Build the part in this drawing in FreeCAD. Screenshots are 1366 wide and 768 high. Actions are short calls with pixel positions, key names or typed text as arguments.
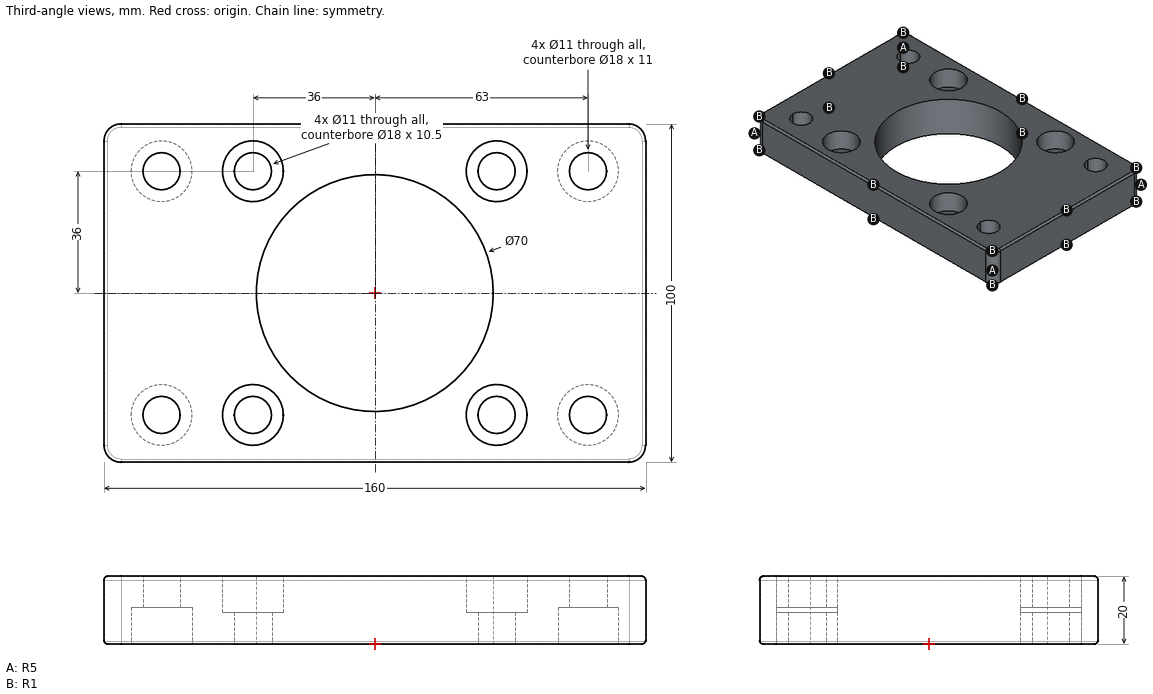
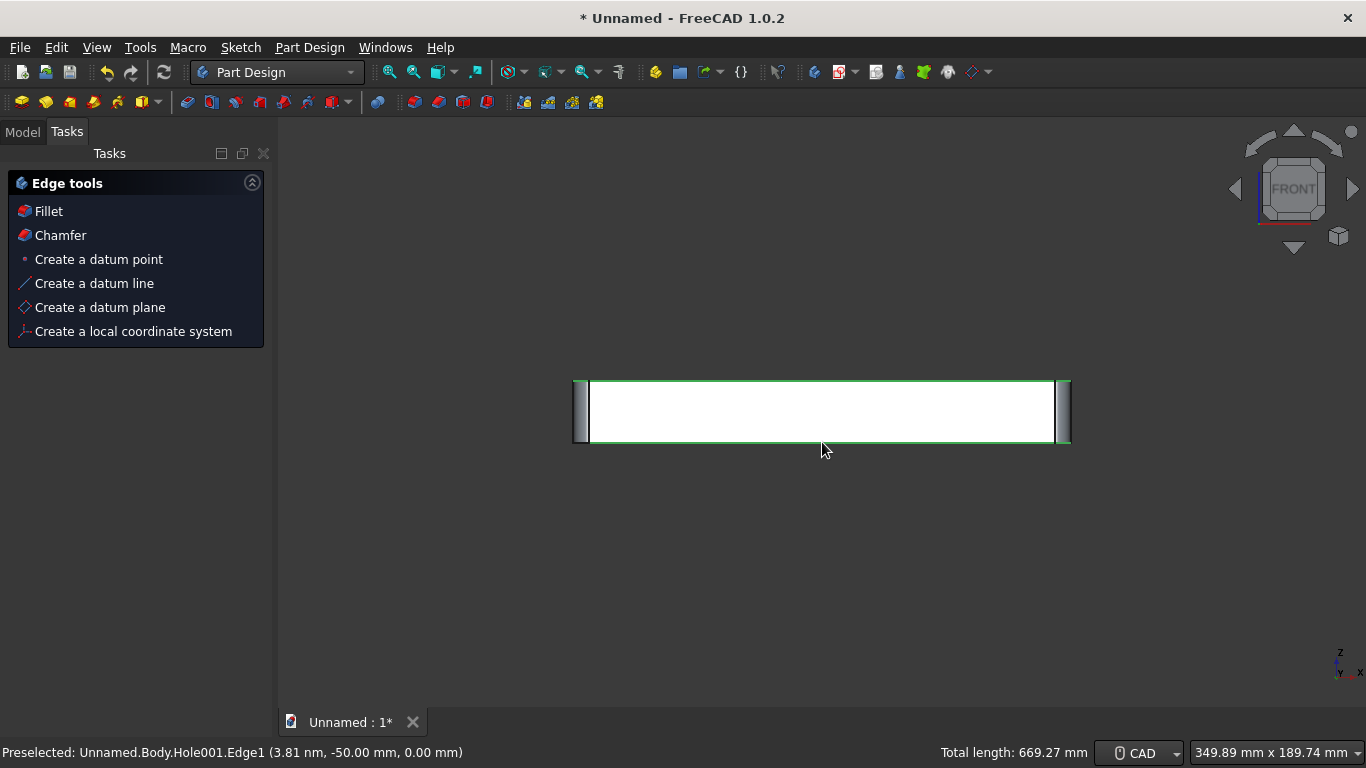
click(578, 442, ctrl)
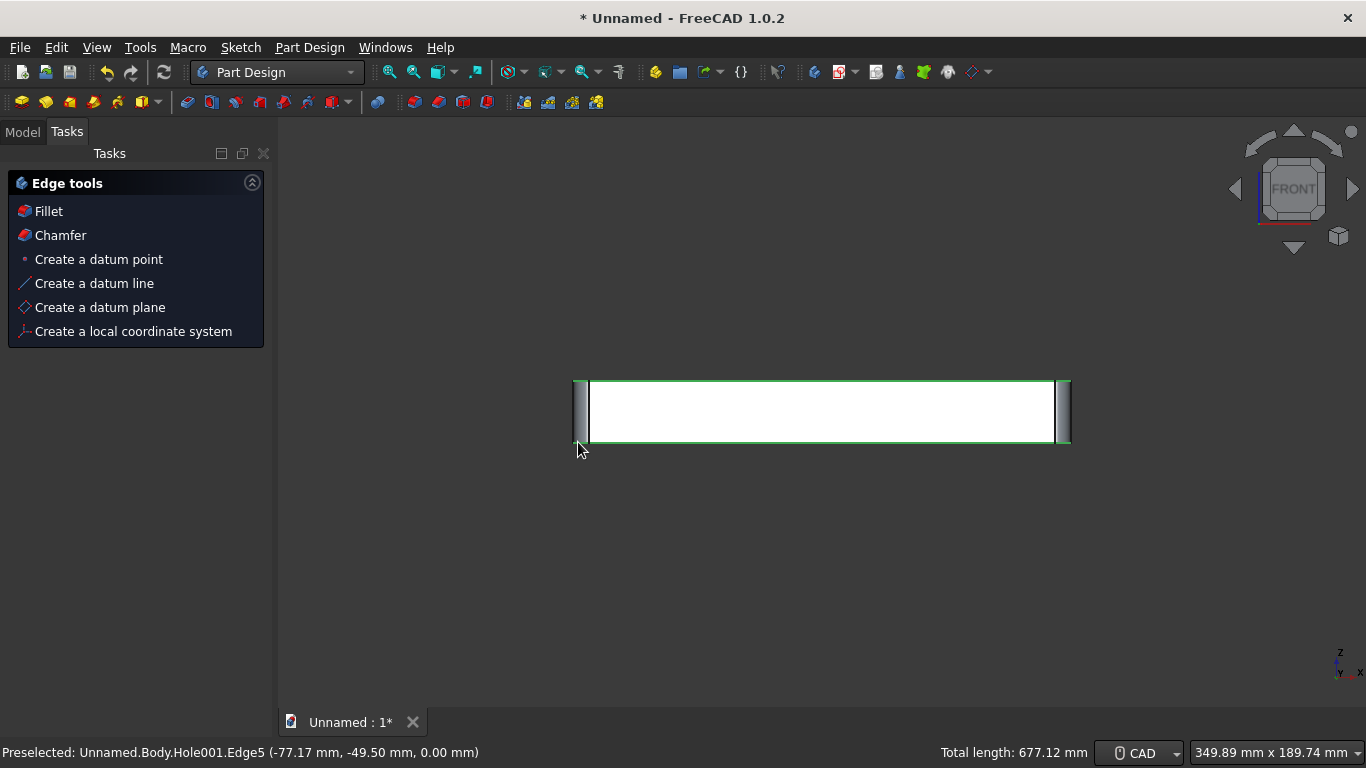
key(3)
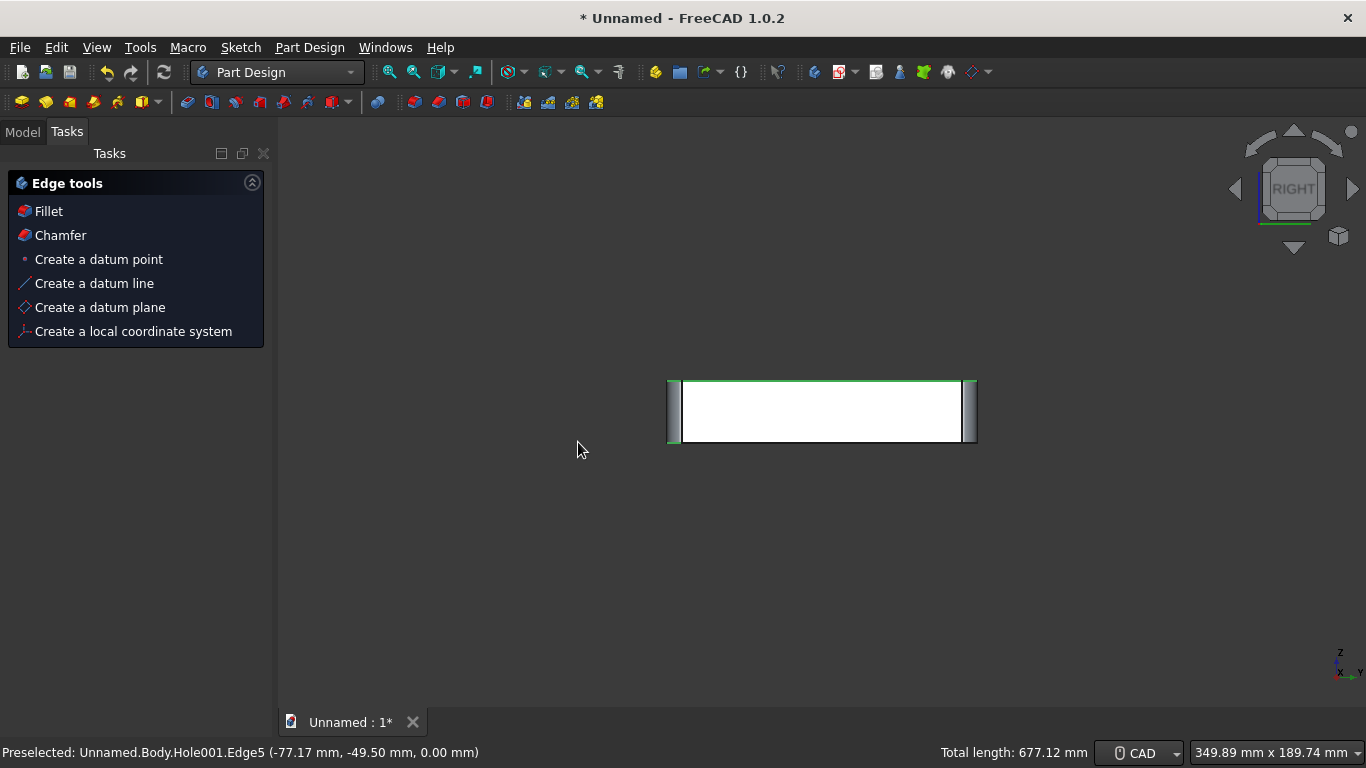
click(390, 72)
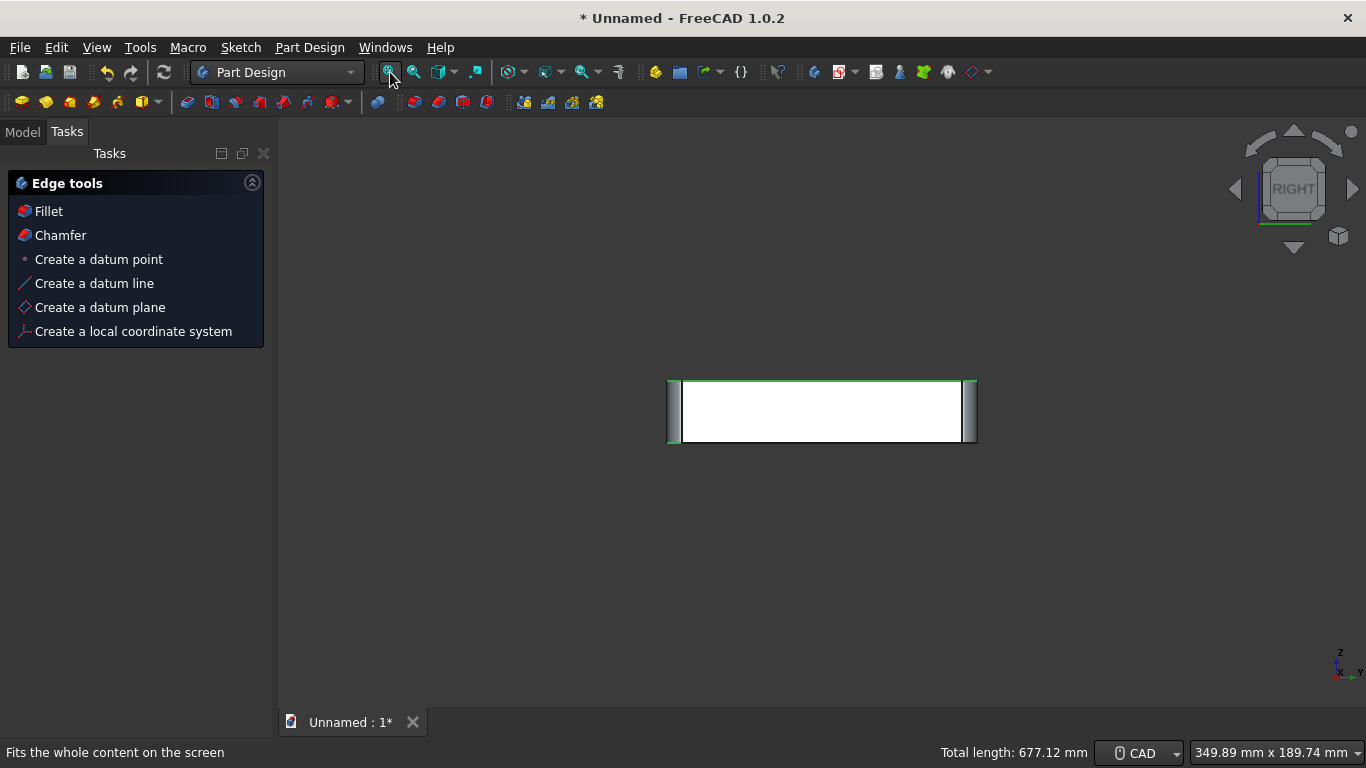
click(822, 442, ctrl)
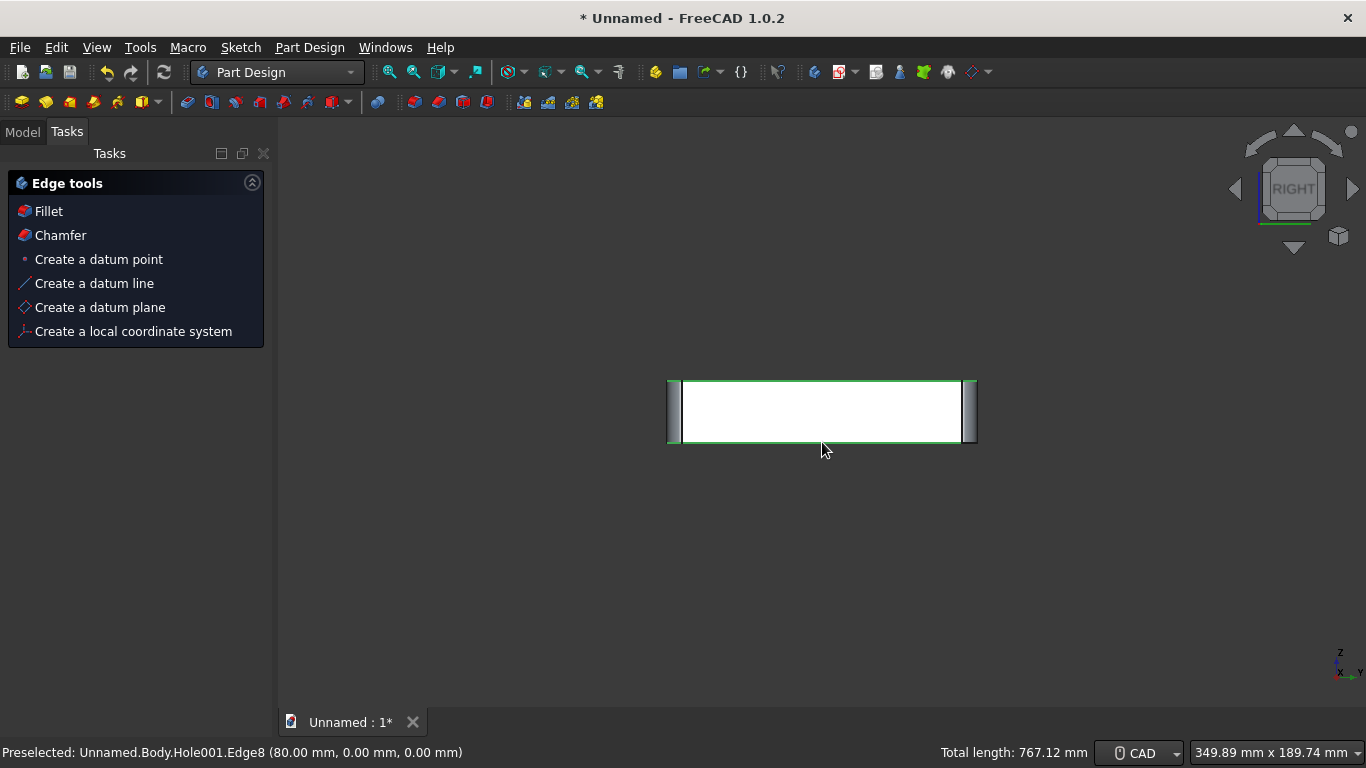
click(973, 442, ctrl)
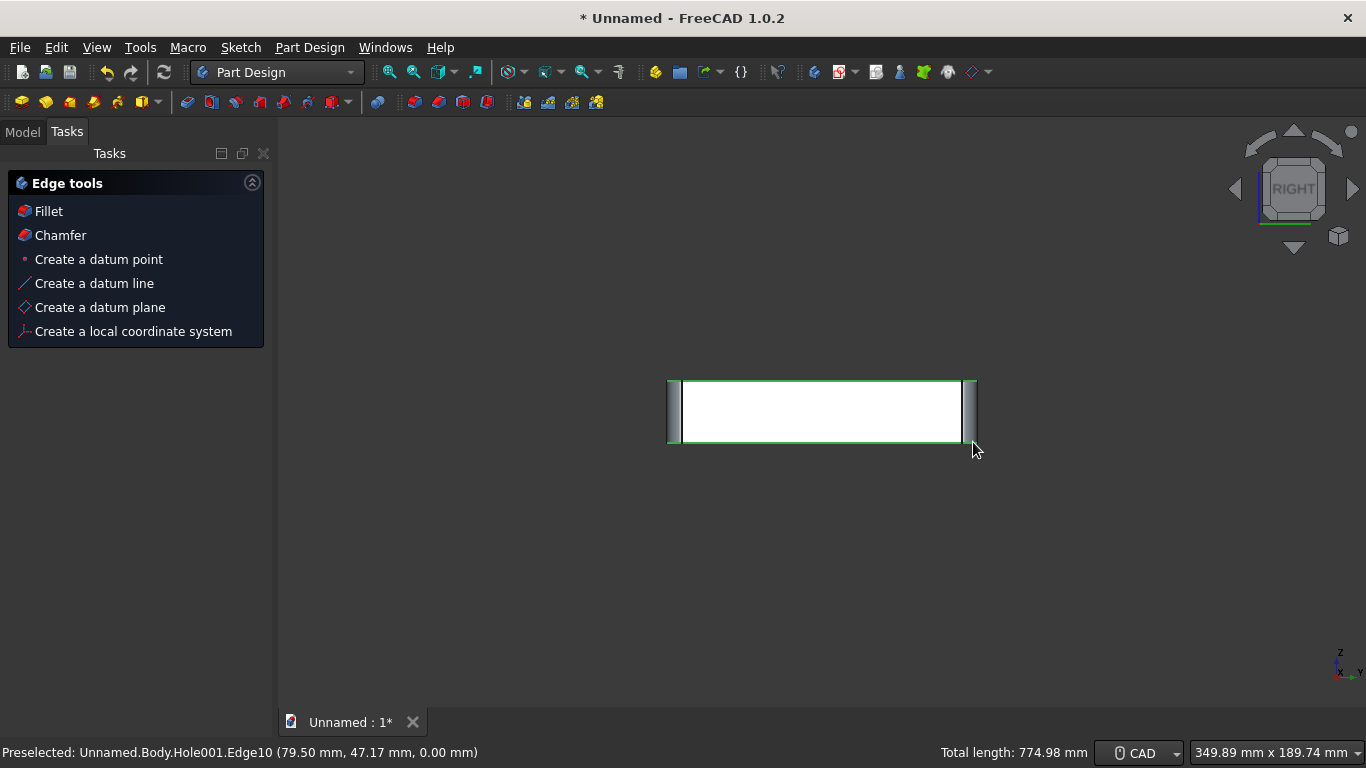
key(5)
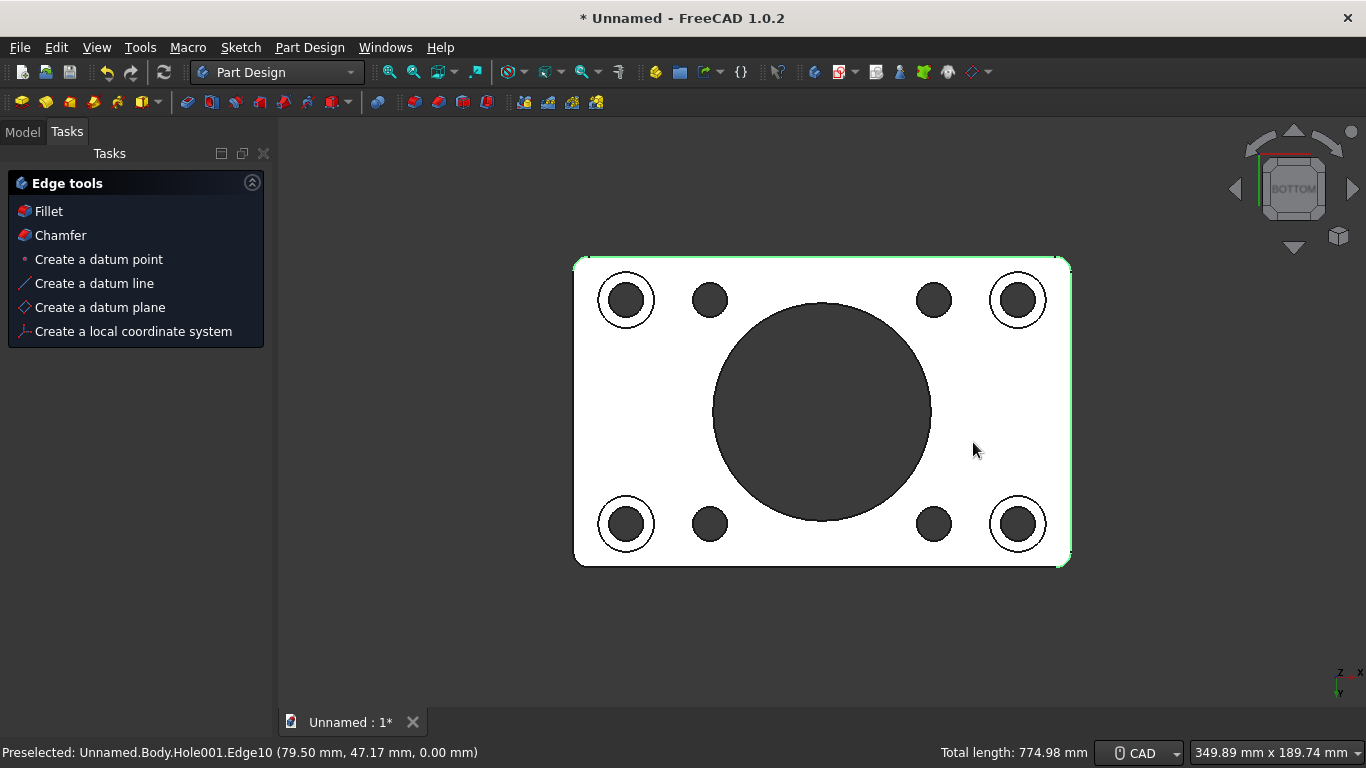
click(573, 411, ctrl)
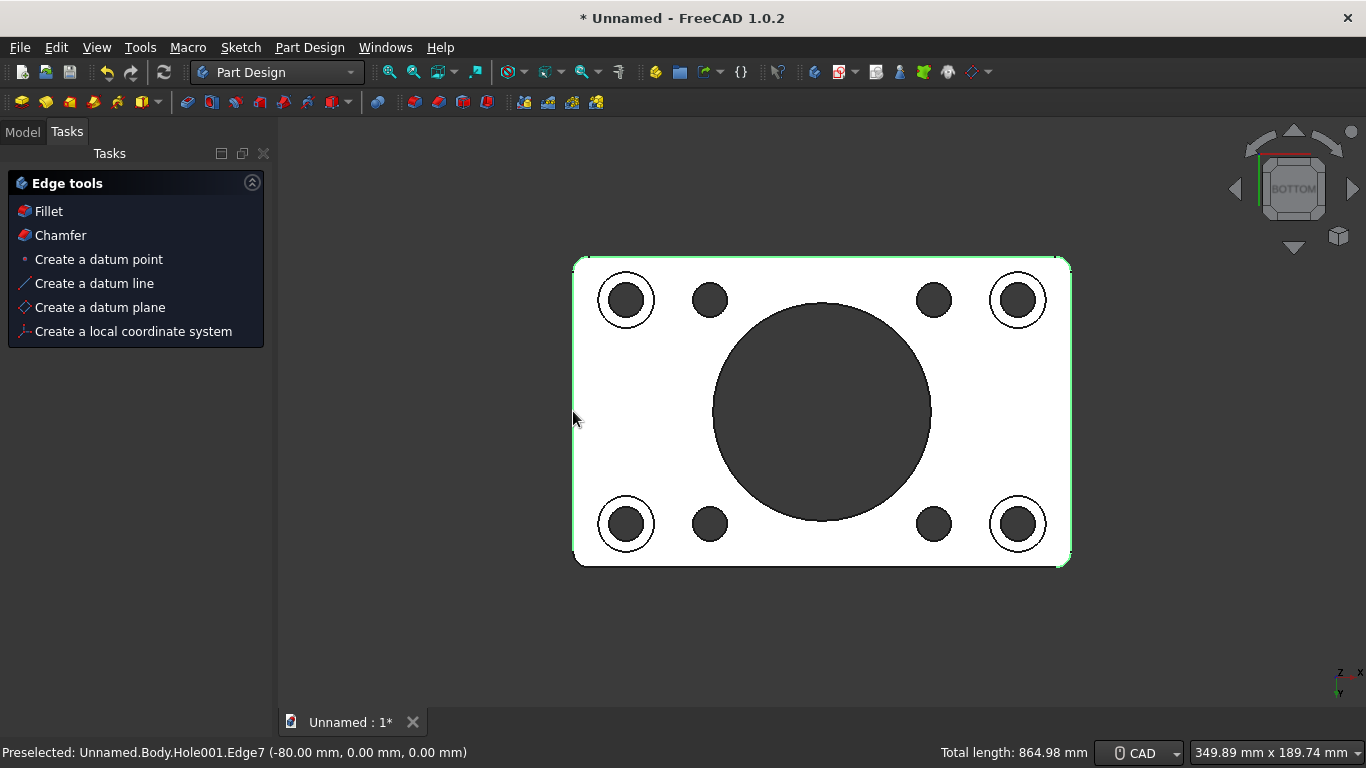
click(822, 566, ctrl)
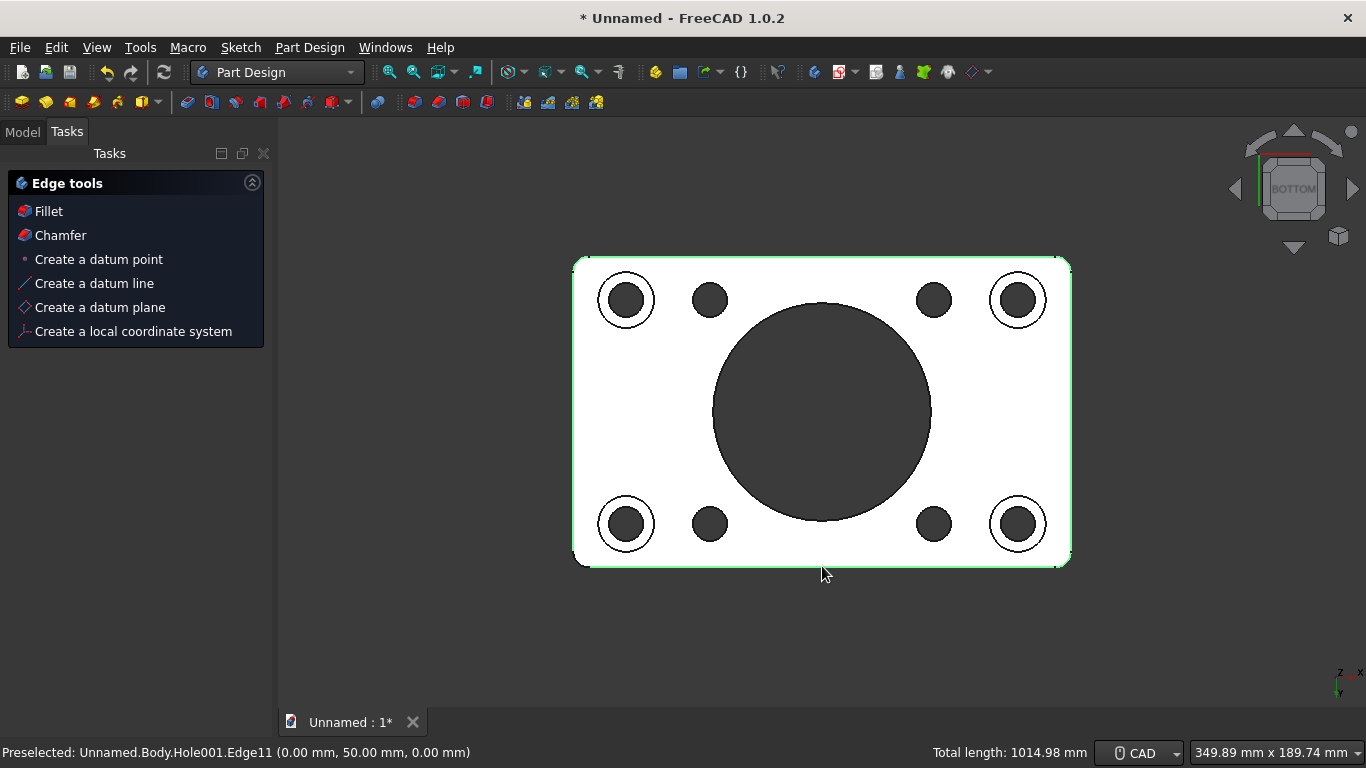
click(578, 562, ctrl)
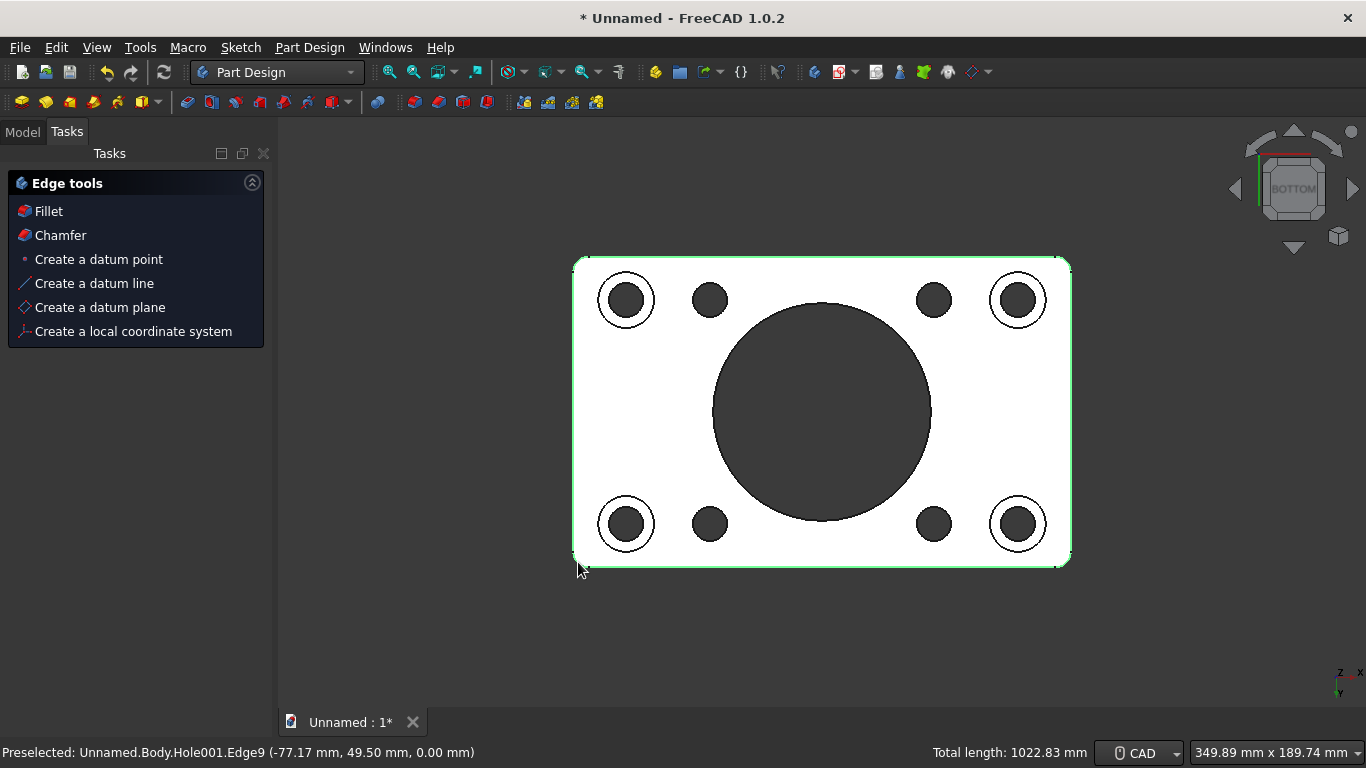
click(416, 102)